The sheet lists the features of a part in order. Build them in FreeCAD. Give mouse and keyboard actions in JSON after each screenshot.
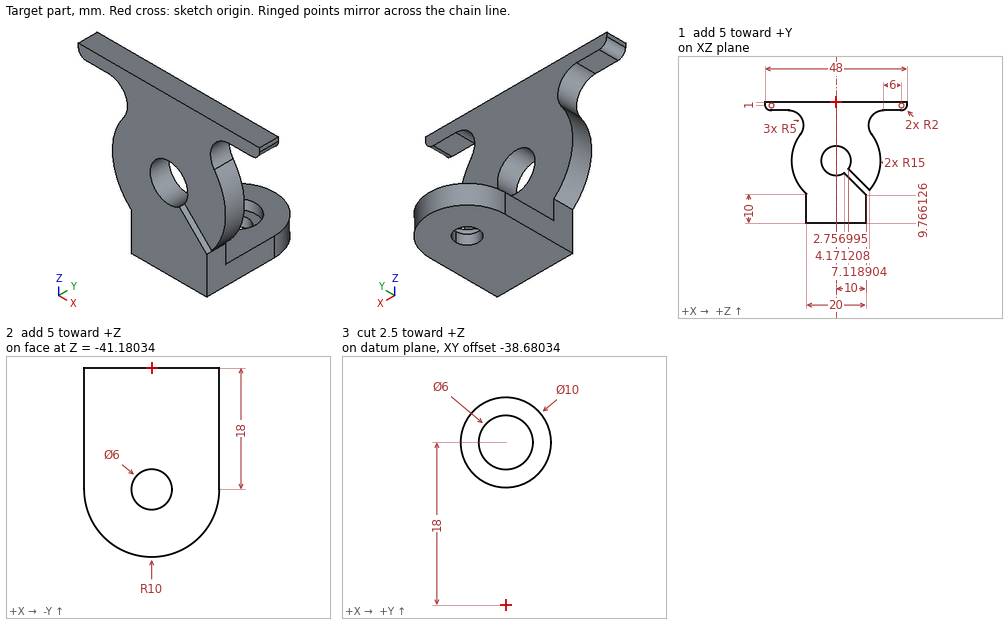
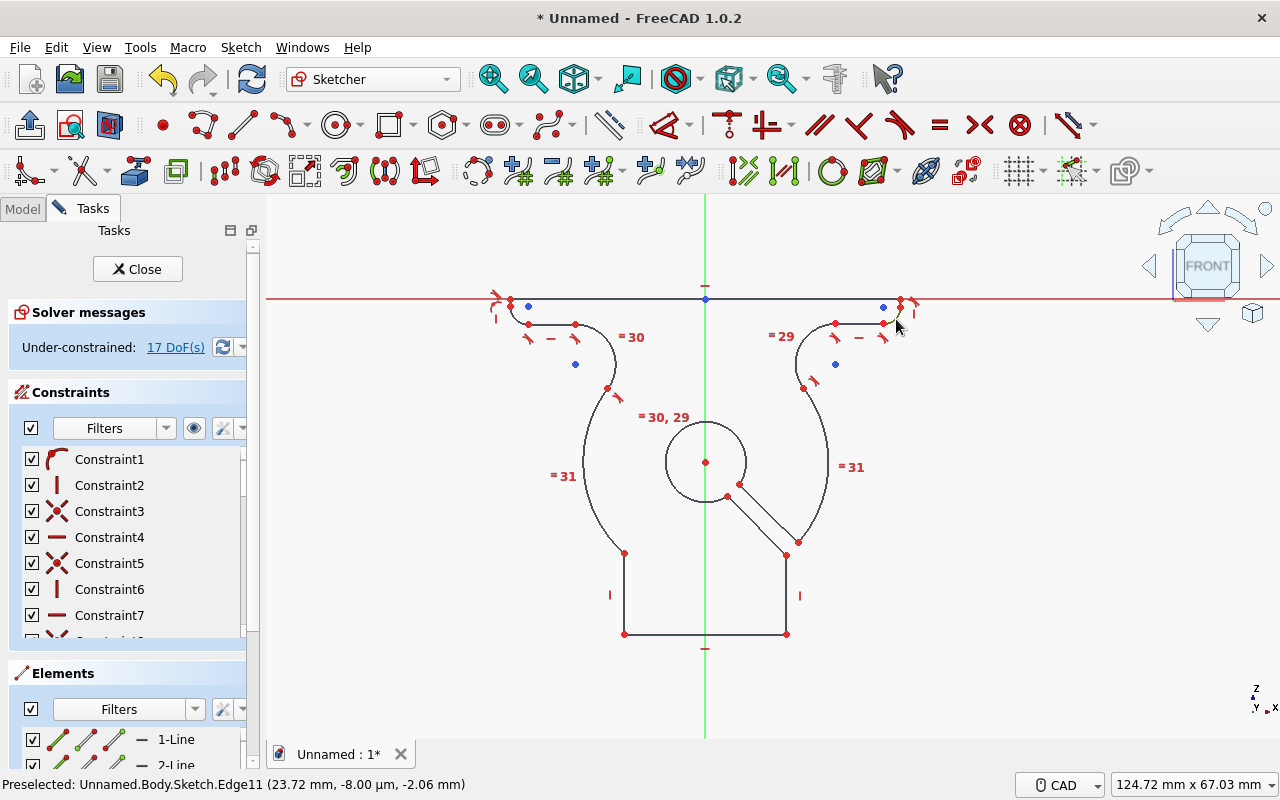
{"action": "left_click", "coordinate": [516, 319]}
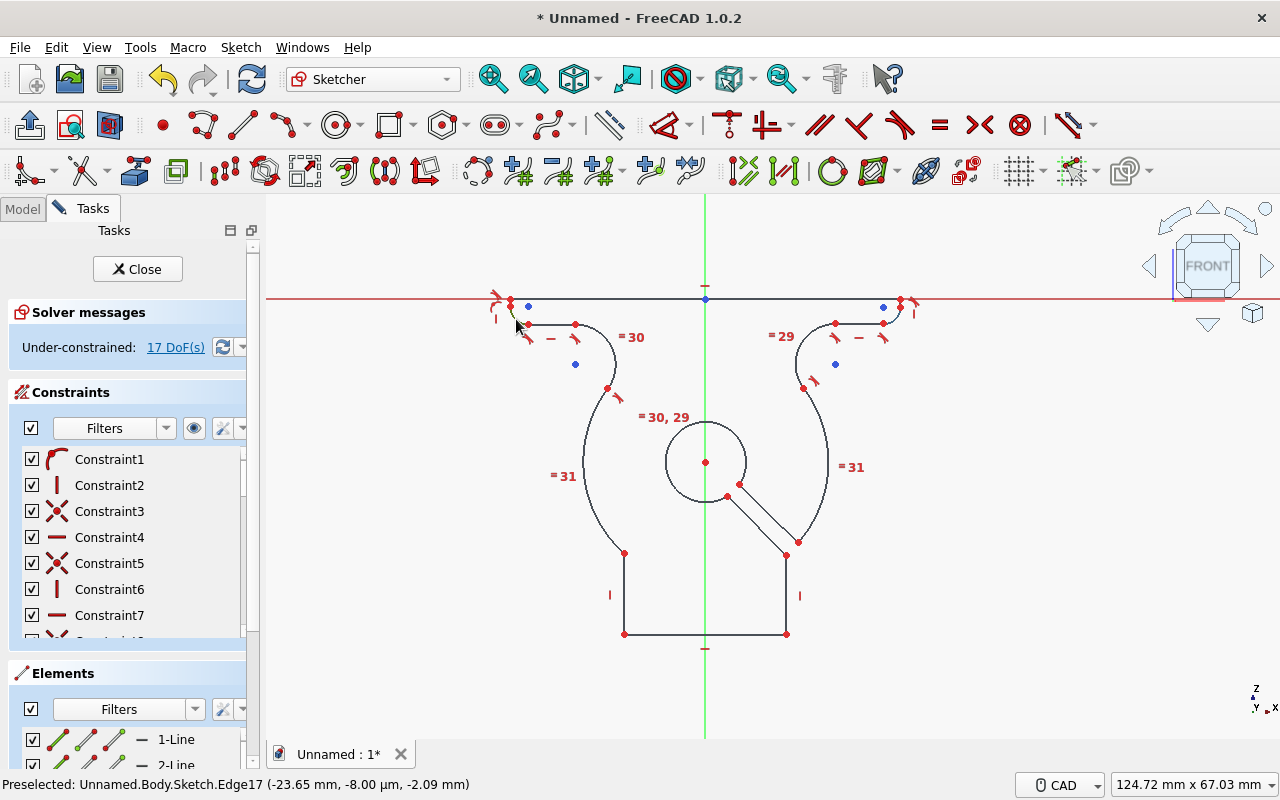
{"action": "key", "text": "e"}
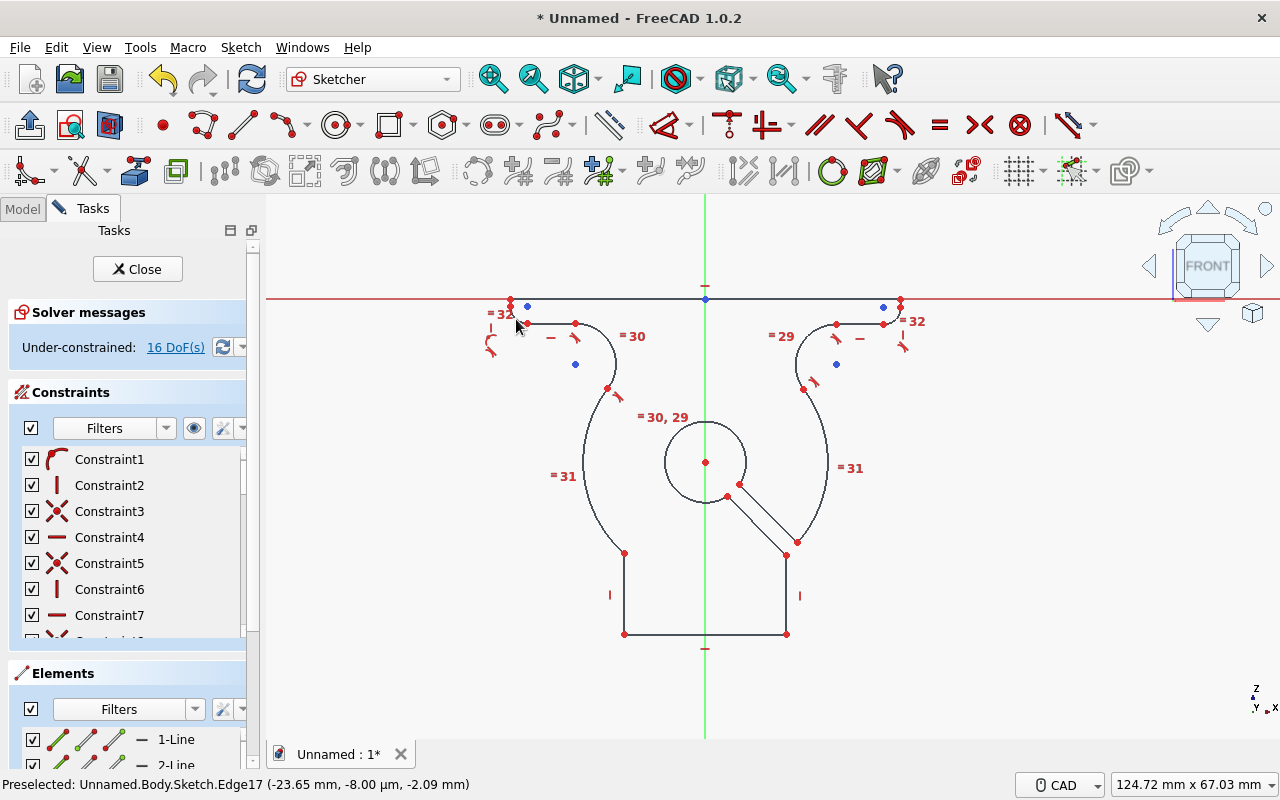
{"action": "left_click", "coordinate": [706, 462]}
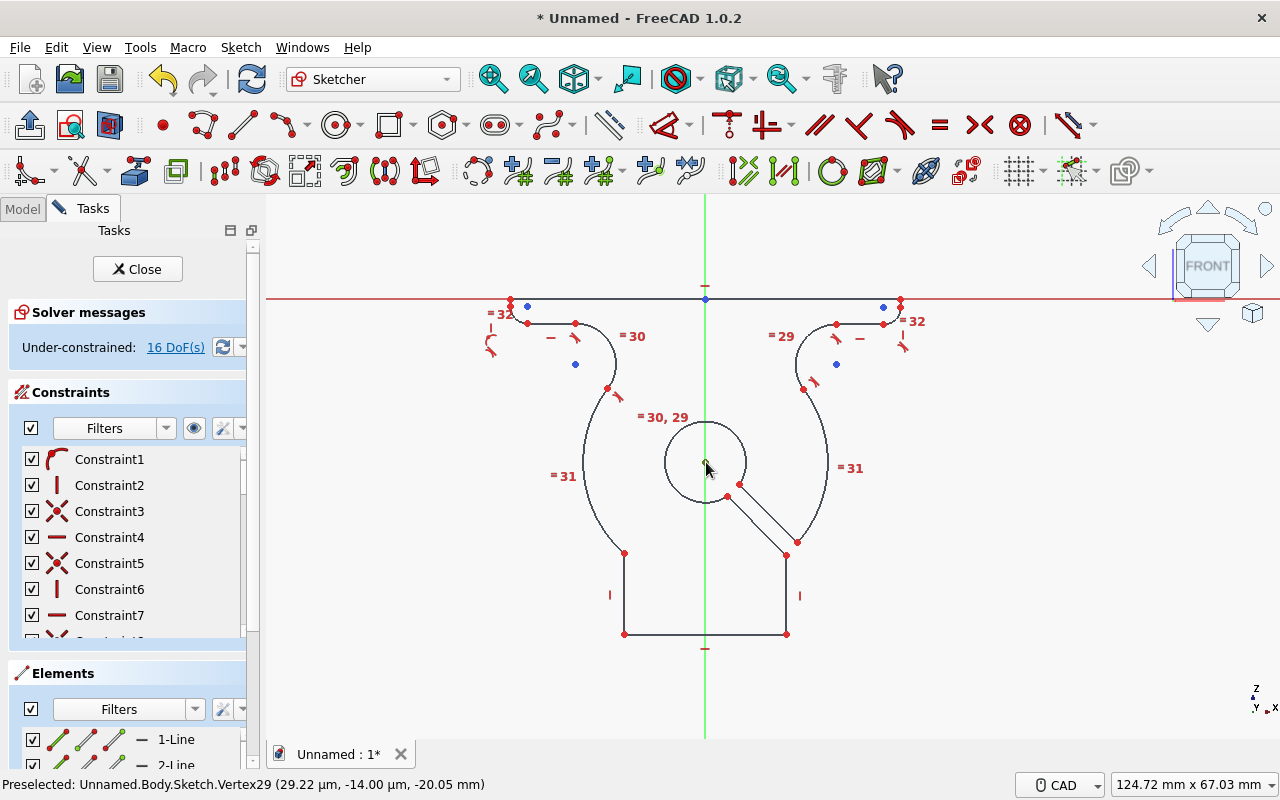
{"action": "left_click", "coordinate": [705, 676]}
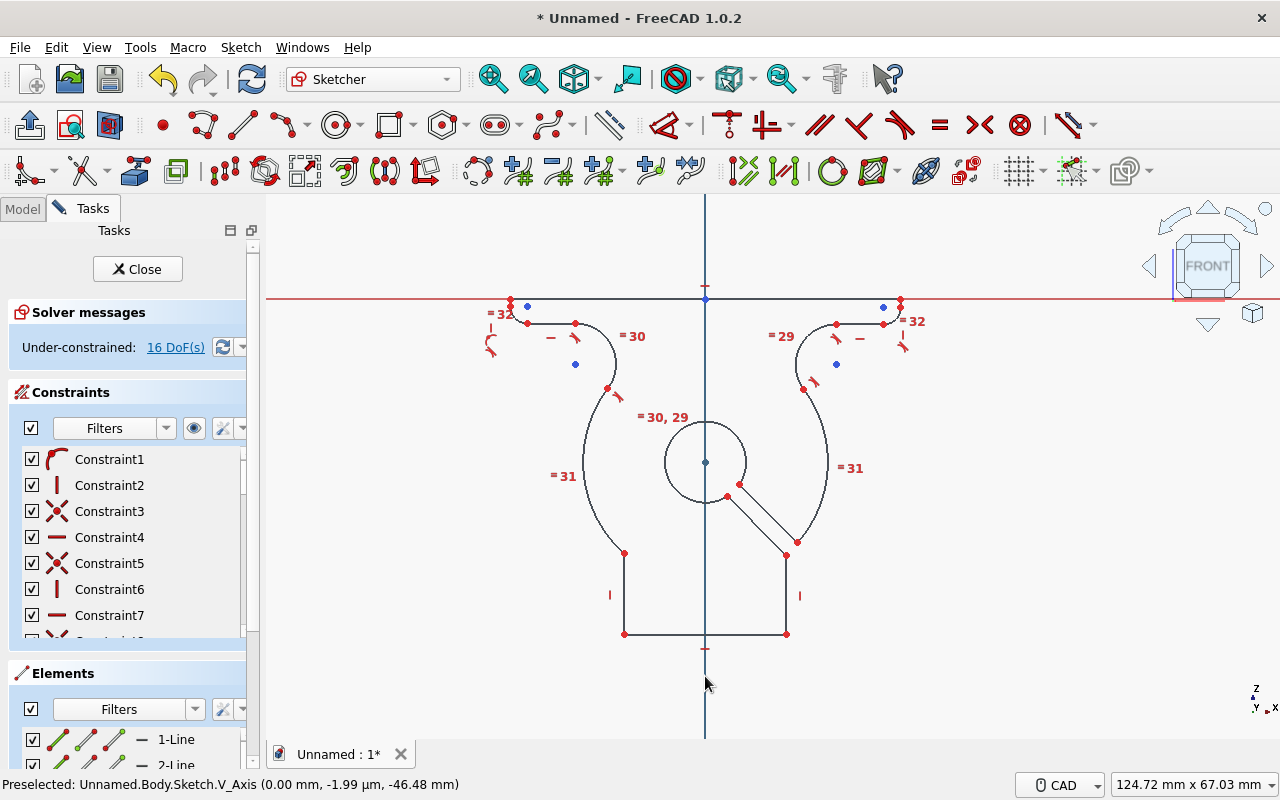
{"action": "left_click", "coordinate": [728, 126]}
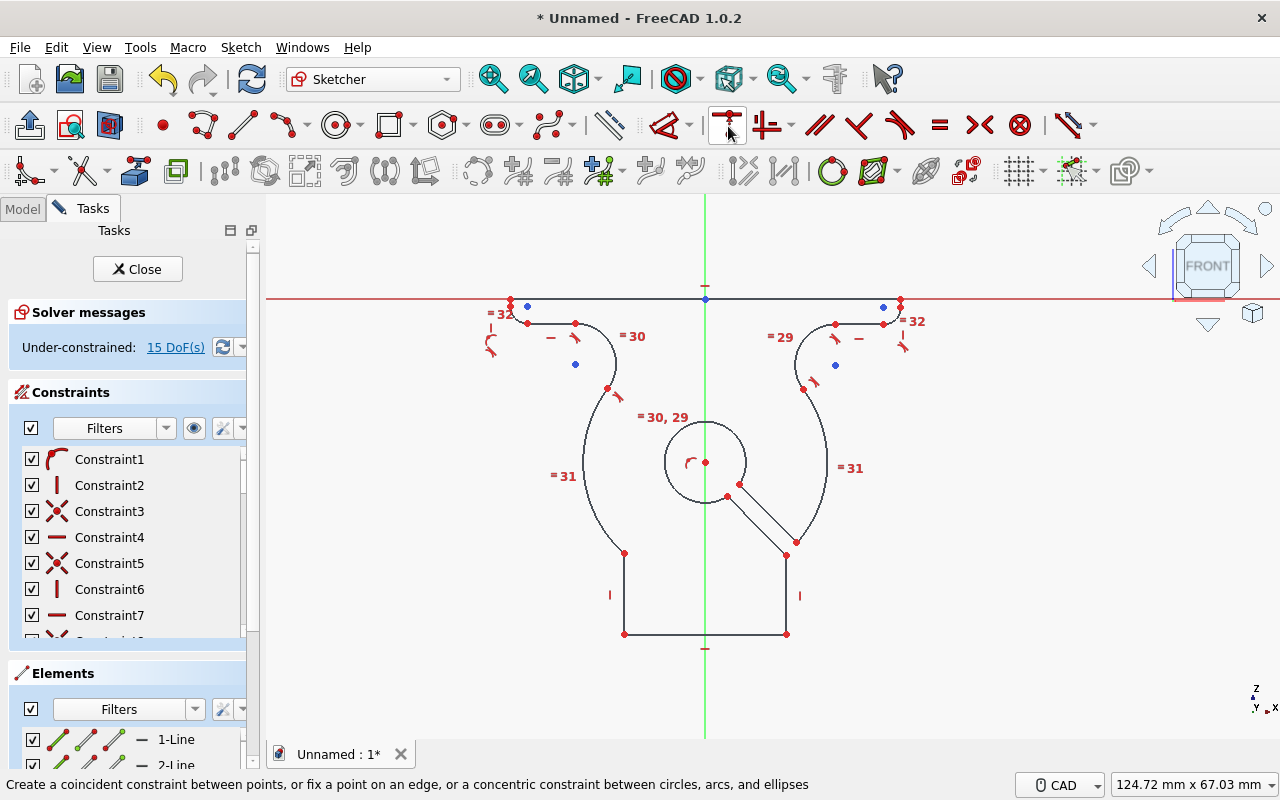
{"action": "left_click", "coordinate": [884, 307]}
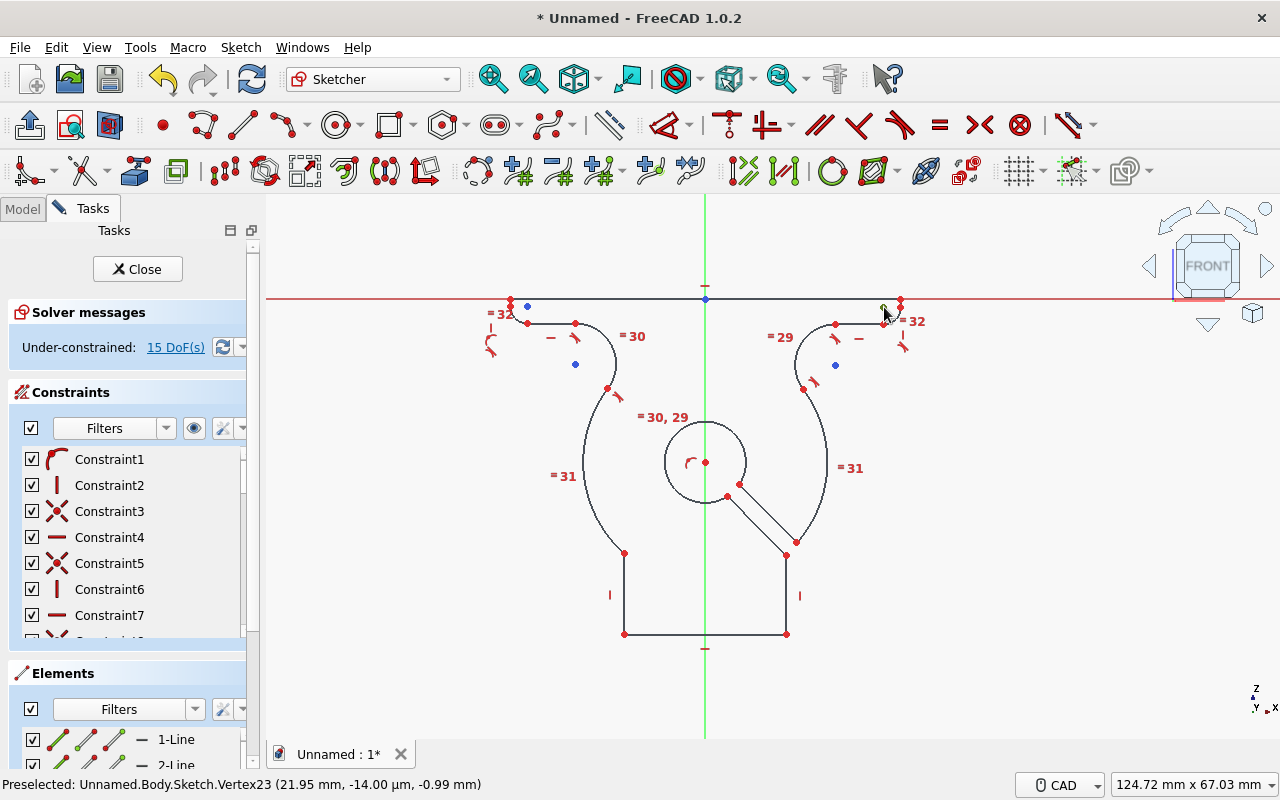
{"action": "left_click", "coordinate": [527, 306]}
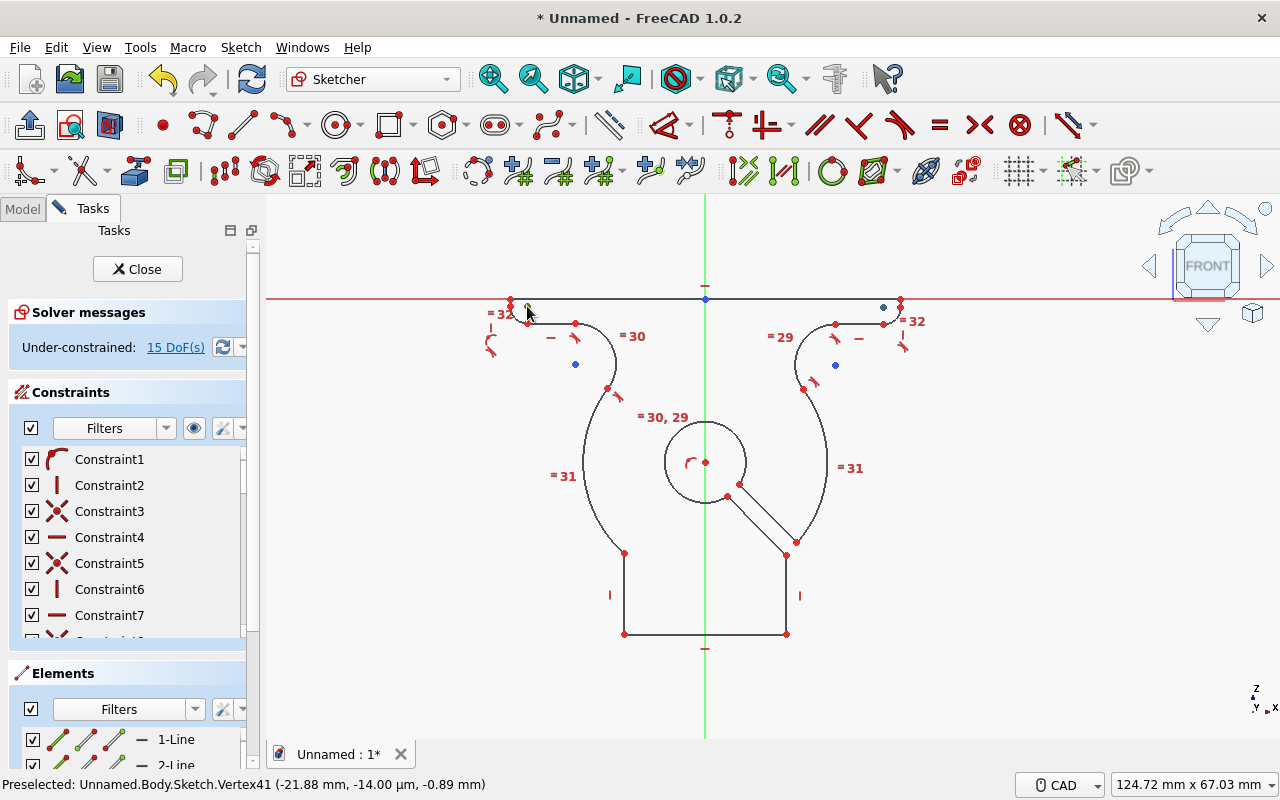
{"action": "left_click", "coordinate": [705, 676]}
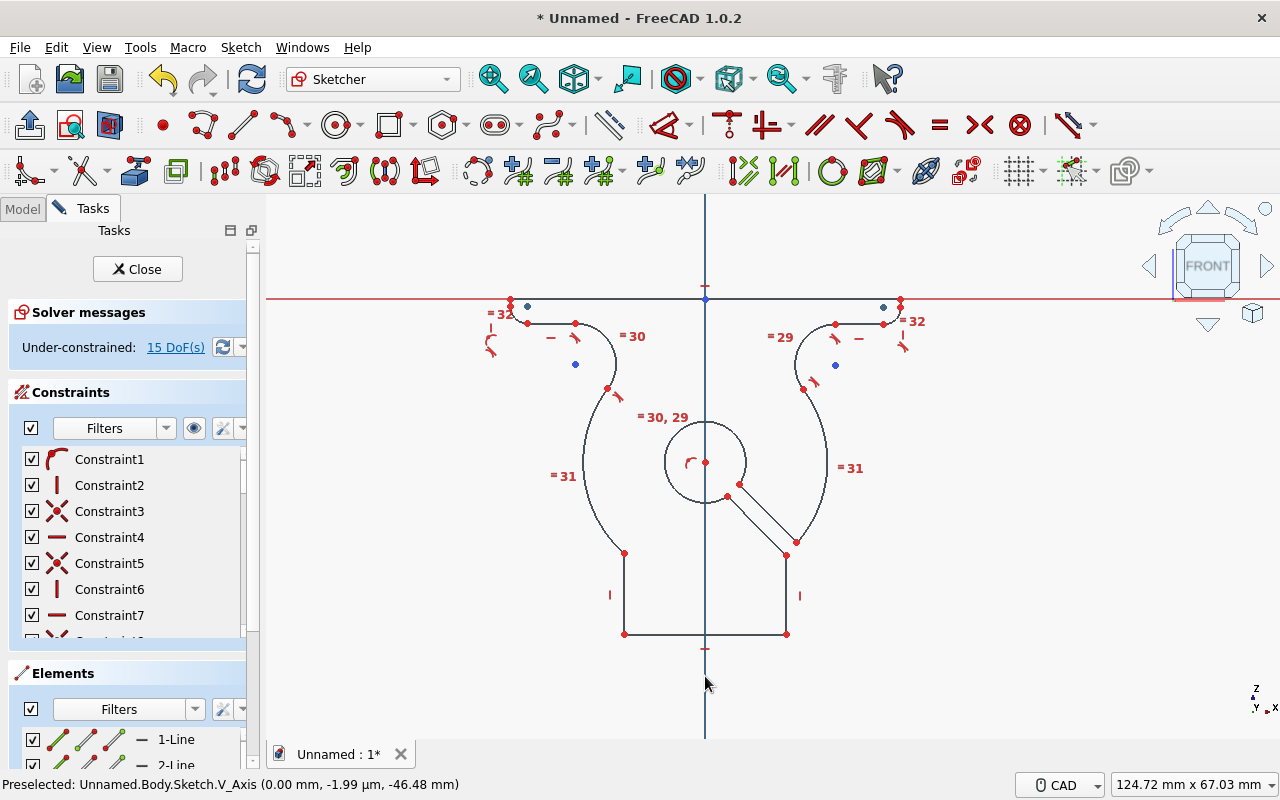
{"action": "left_click", "coordinate": [980, 126]}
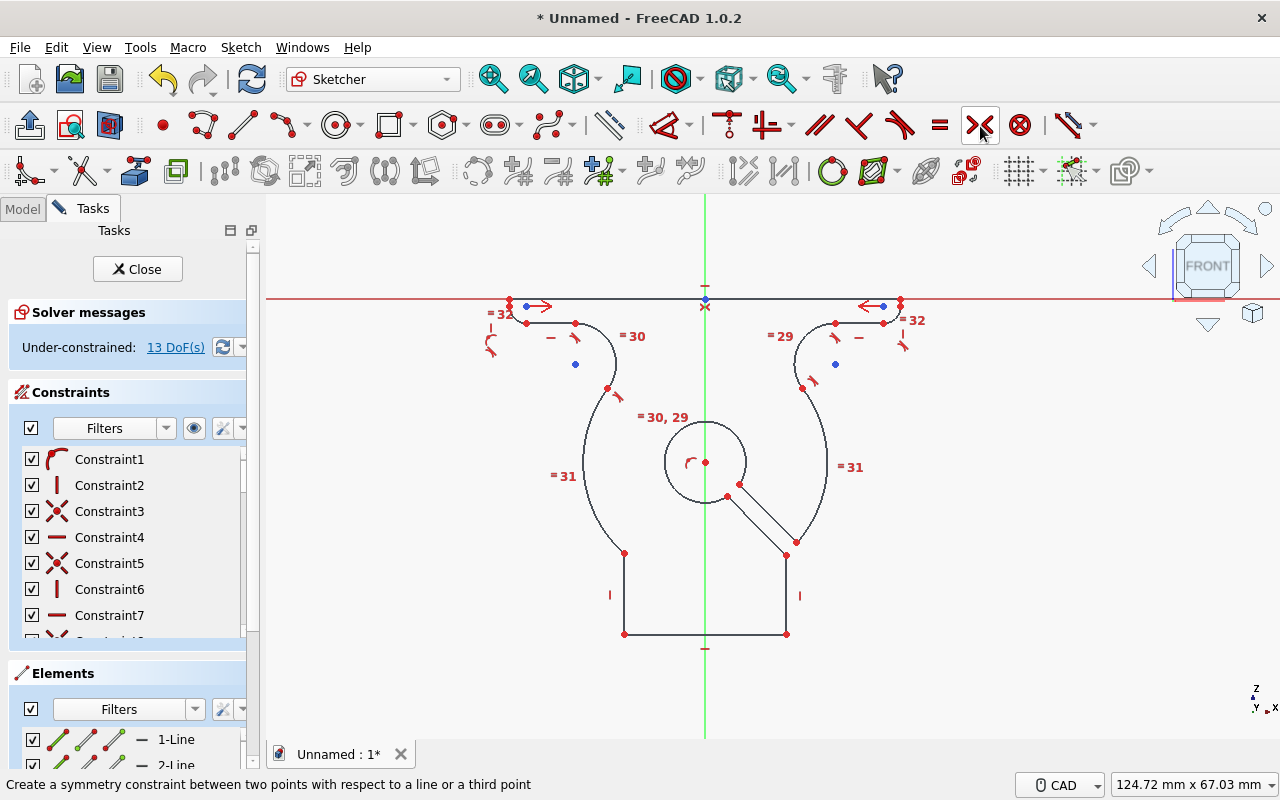
{"action": "scroll", "coordinate": [896, 318], "scroll_direction": "up", "scroll_amount": 5}